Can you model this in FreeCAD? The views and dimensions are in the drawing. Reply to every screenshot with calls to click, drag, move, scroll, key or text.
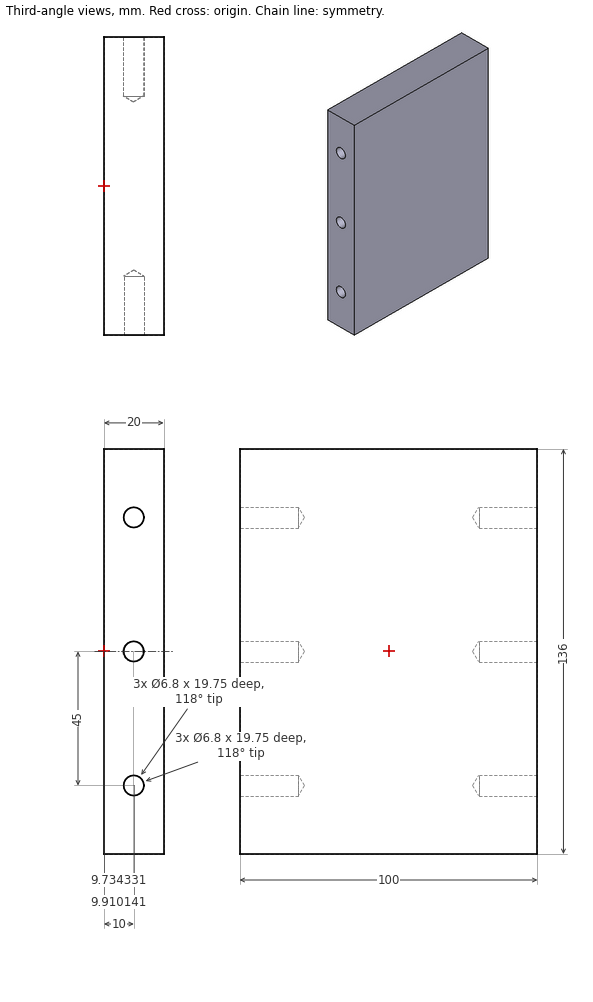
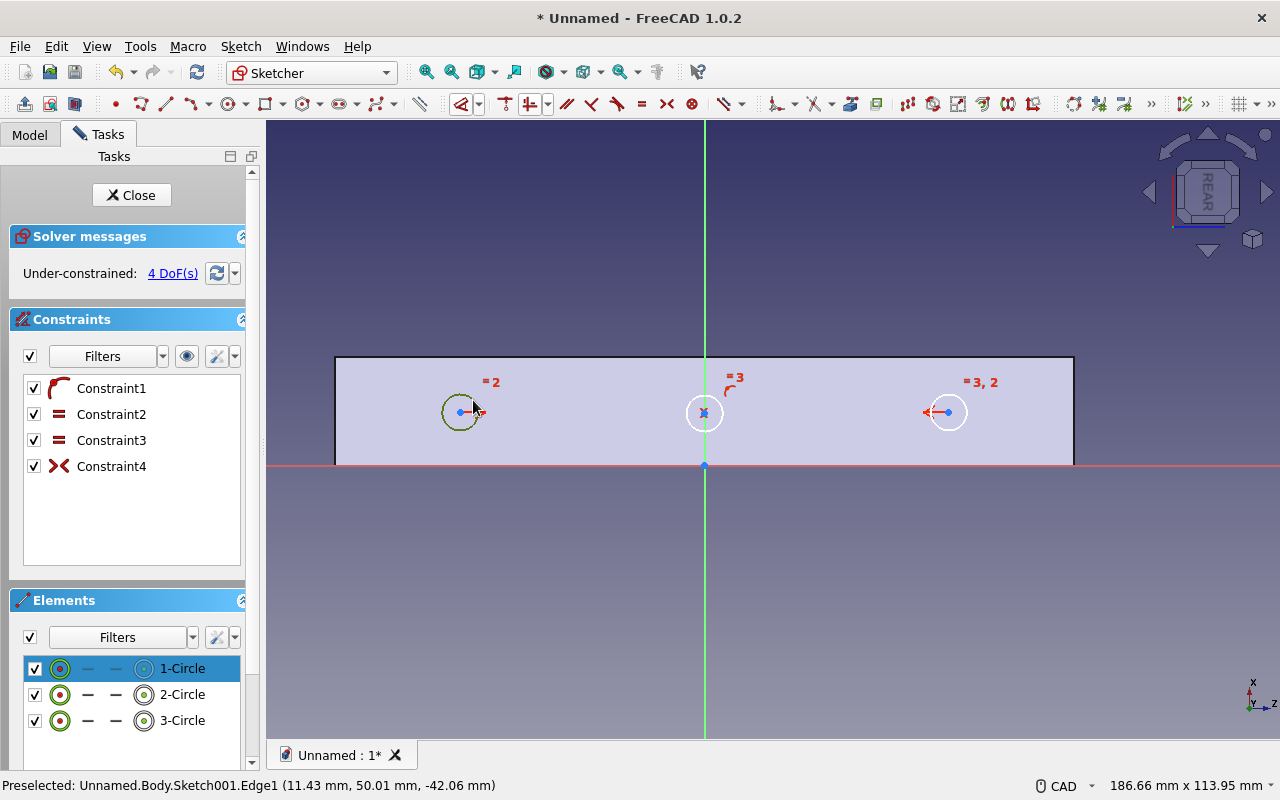
click(478, 104)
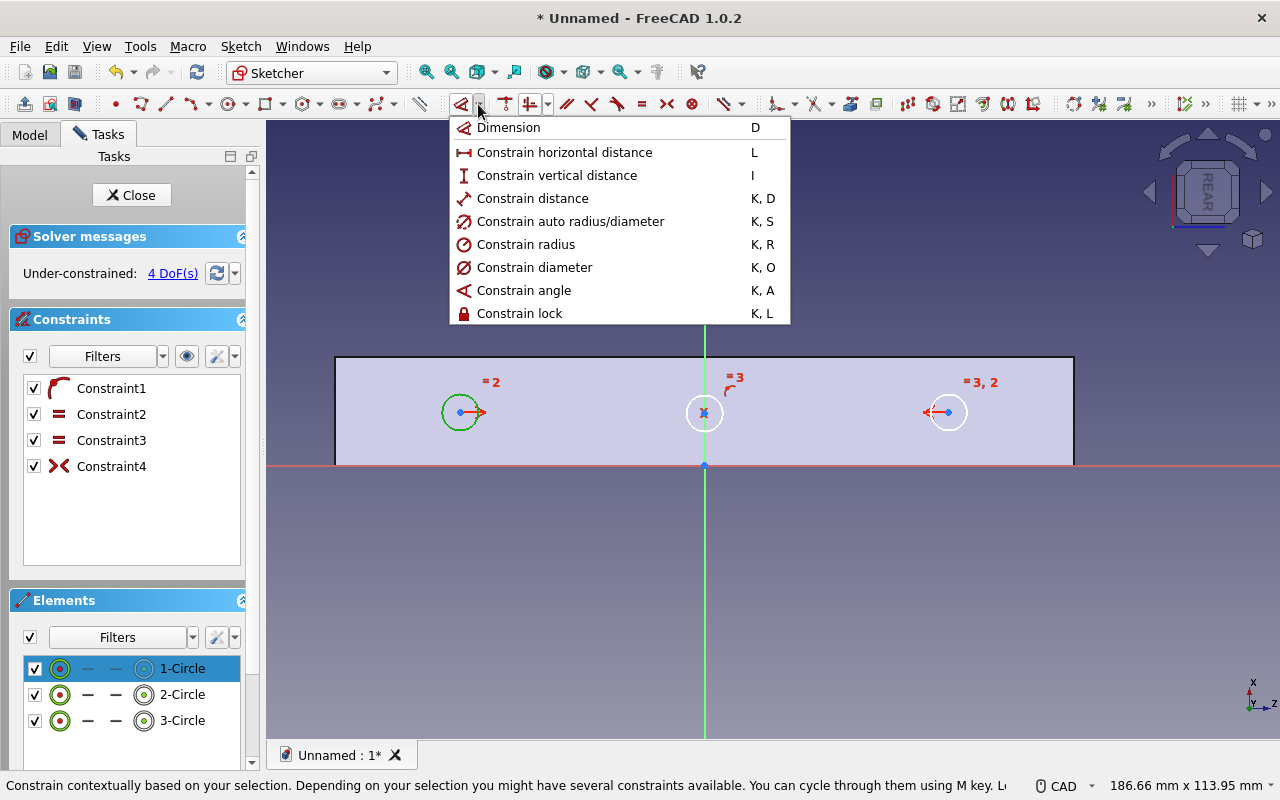
click(620, 268)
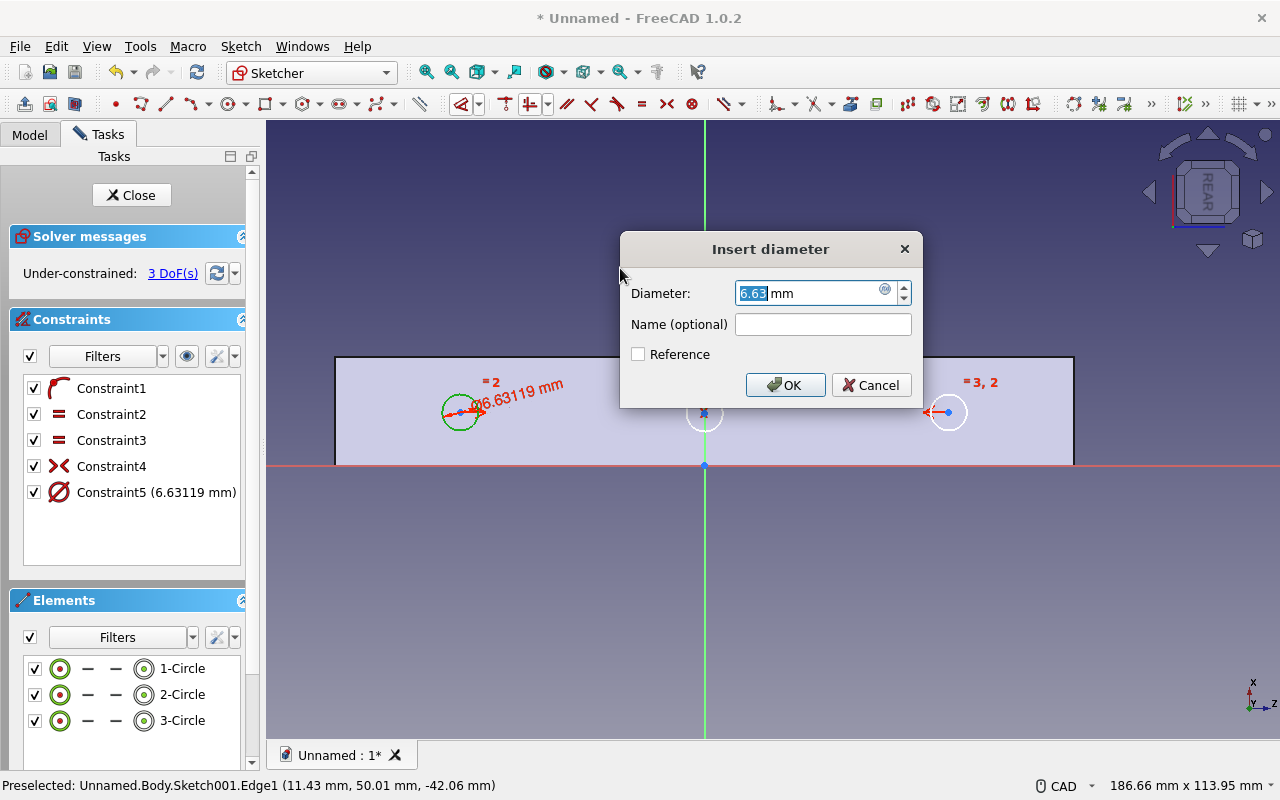
text(6.8)
key(Return)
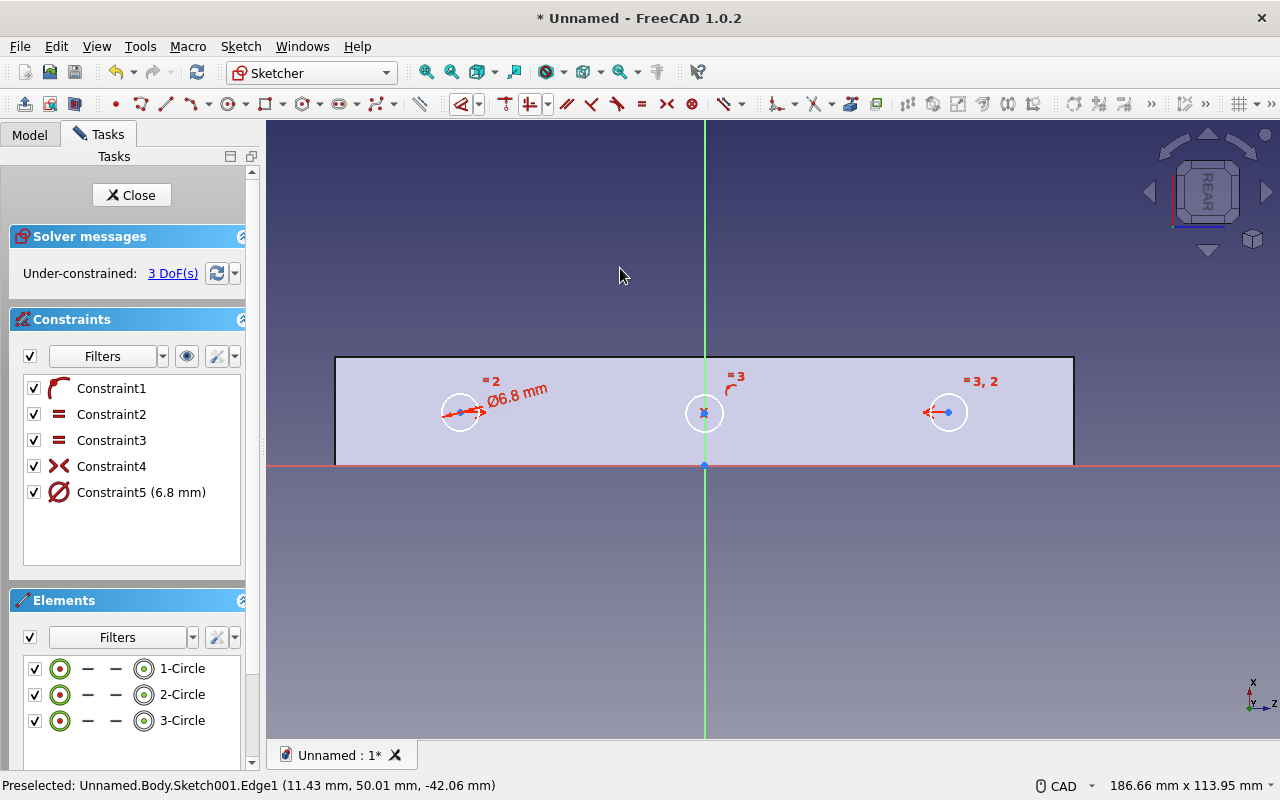
click(460, 412)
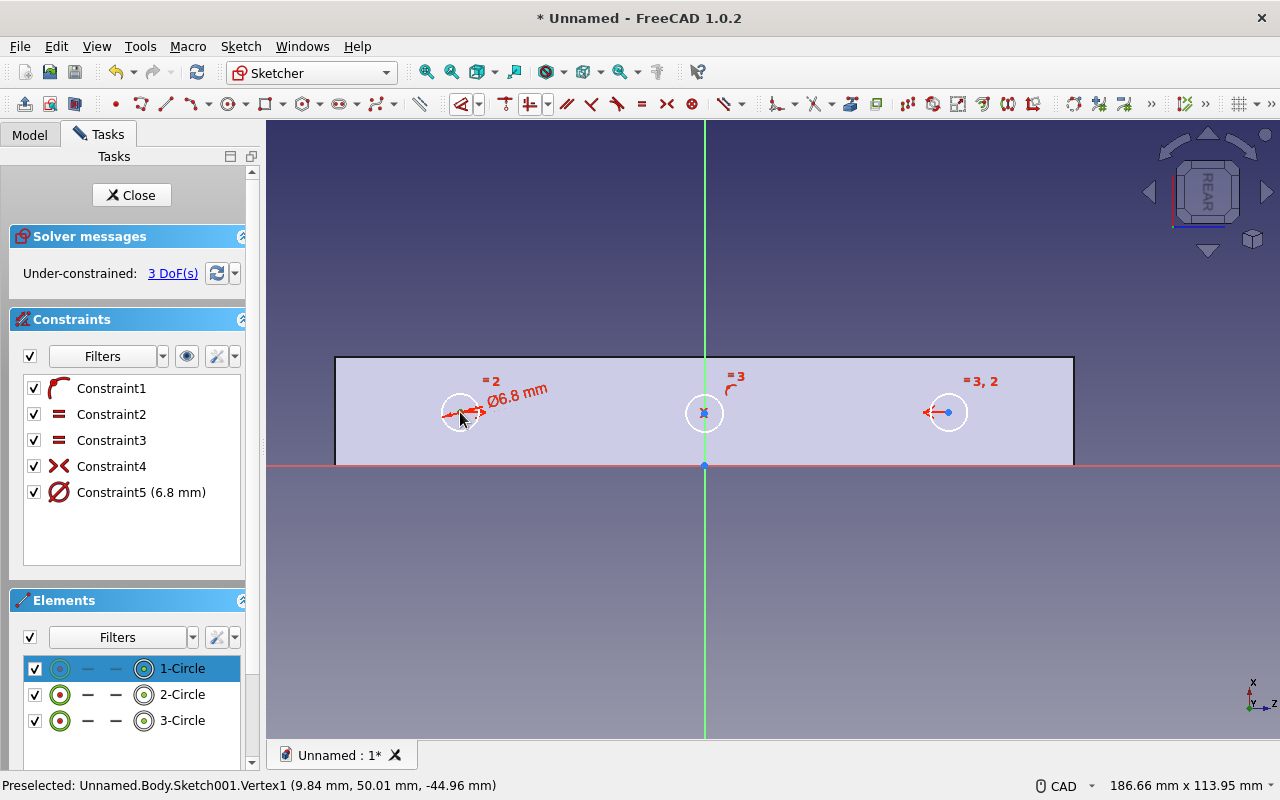
key(l)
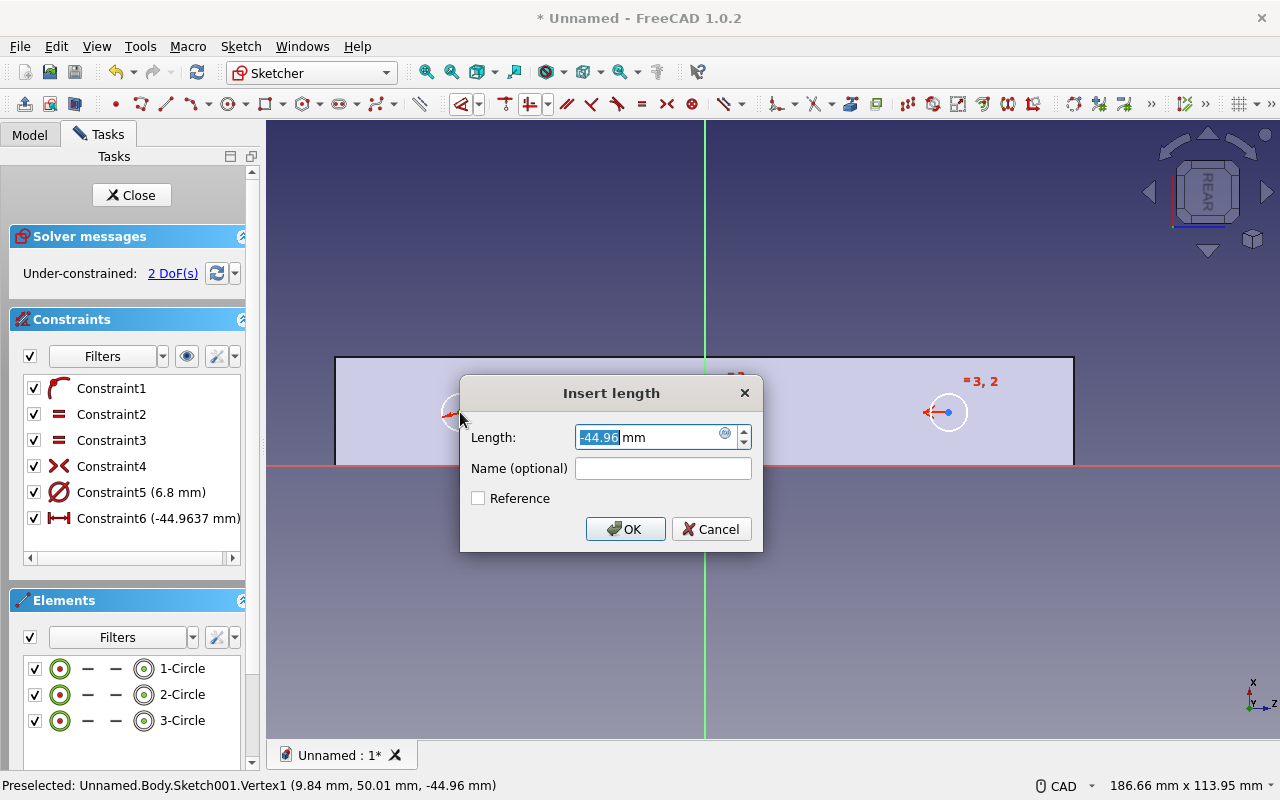
text(-45)
key(Return)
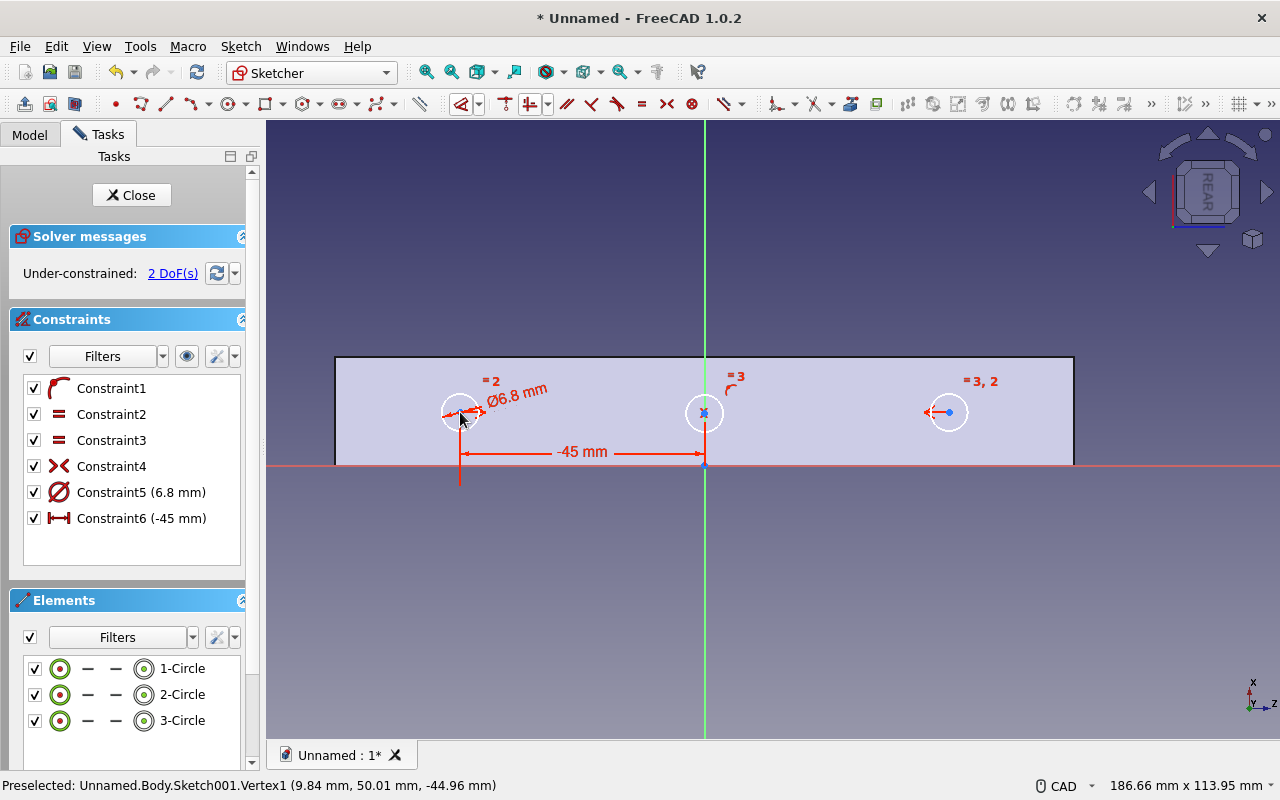
click(460, 412)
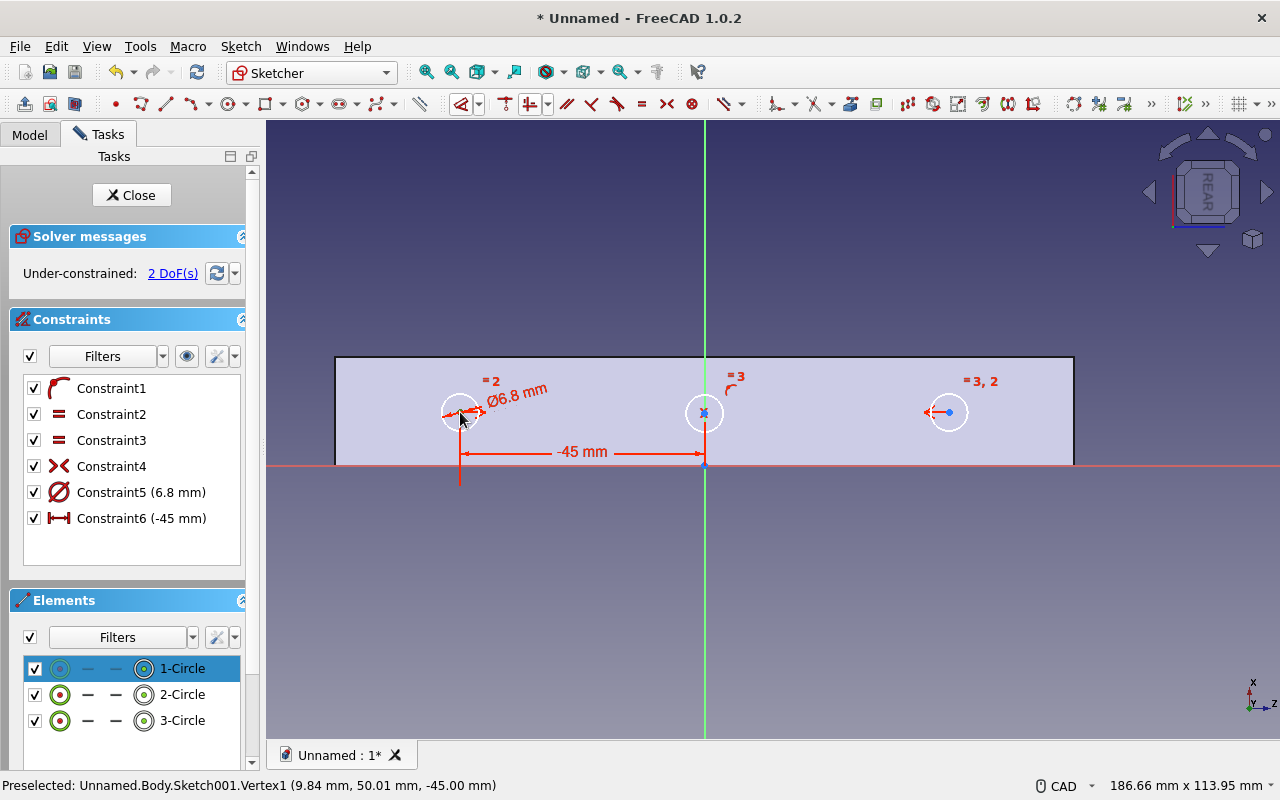
key(i)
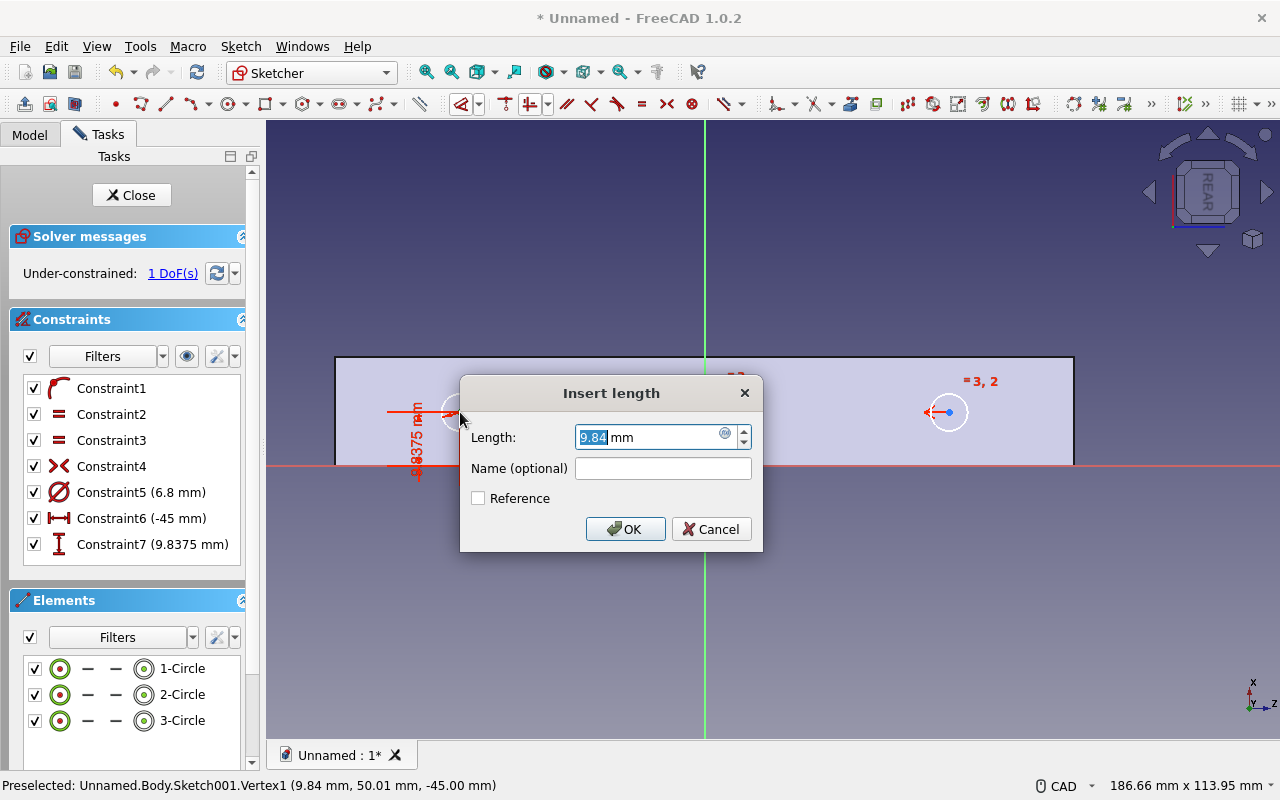
text(9.910141)
key(Return)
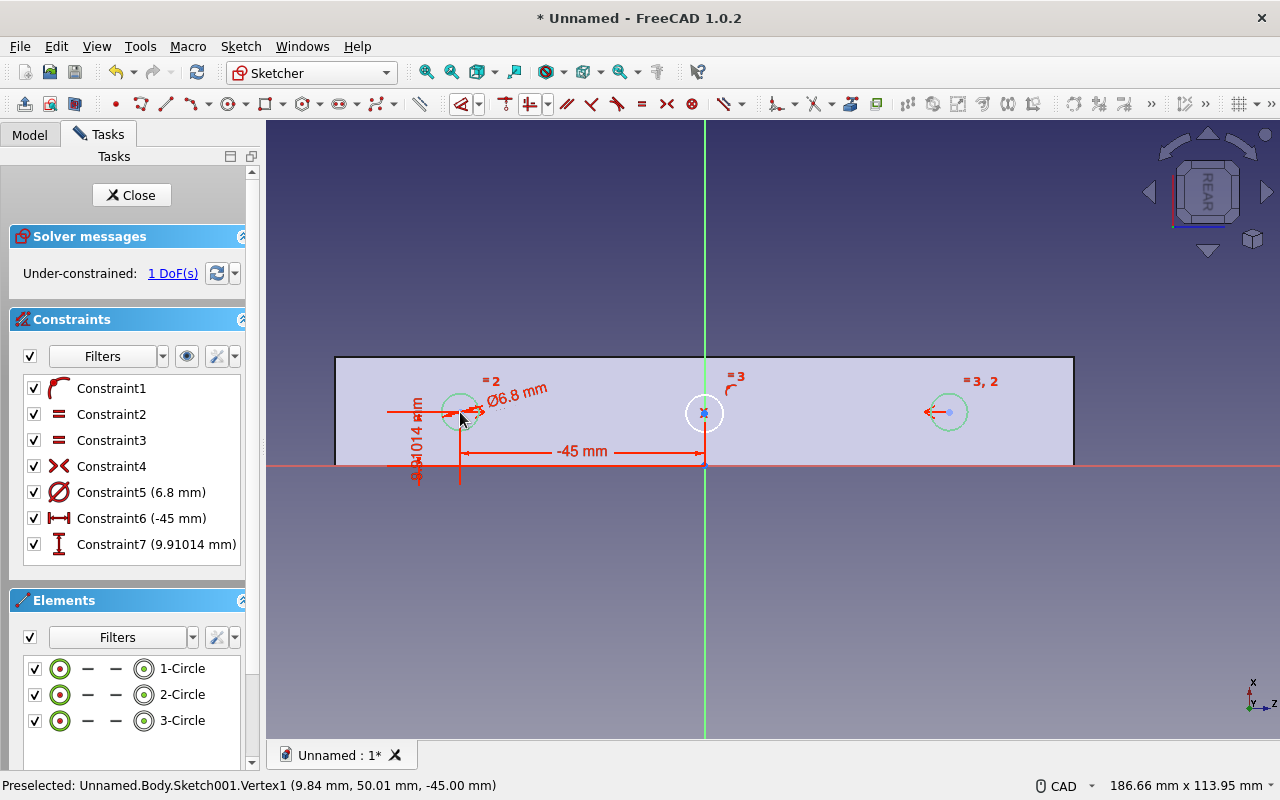
click(705, 413)